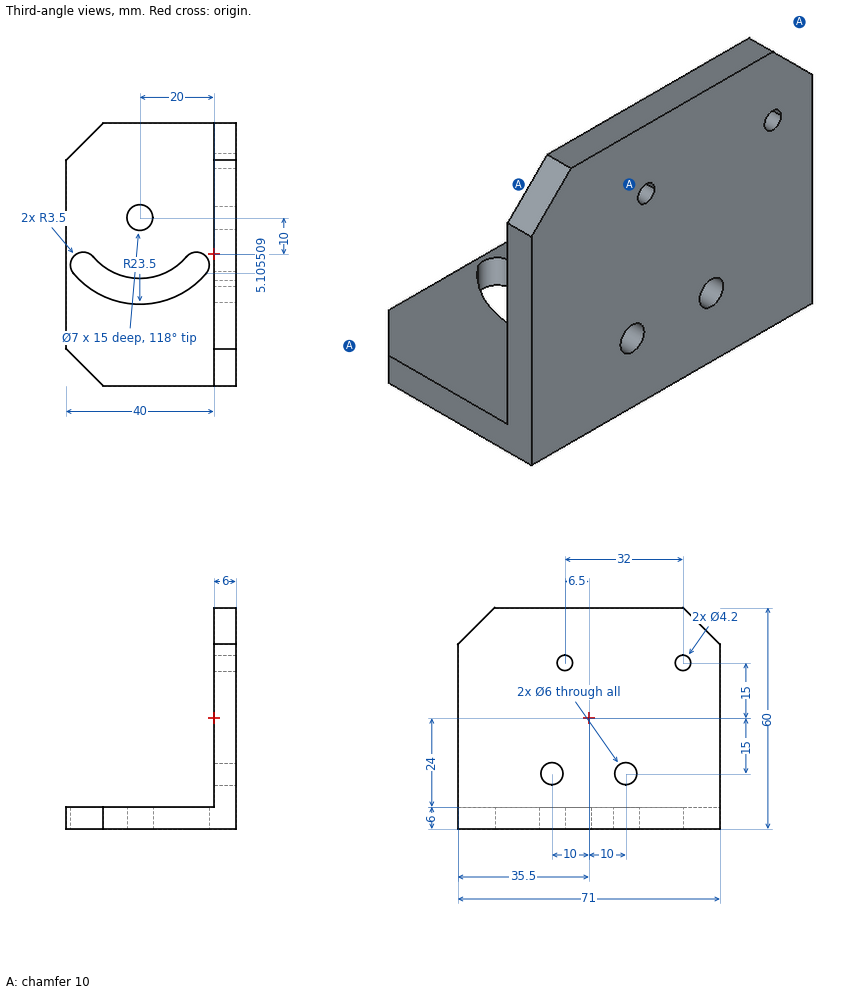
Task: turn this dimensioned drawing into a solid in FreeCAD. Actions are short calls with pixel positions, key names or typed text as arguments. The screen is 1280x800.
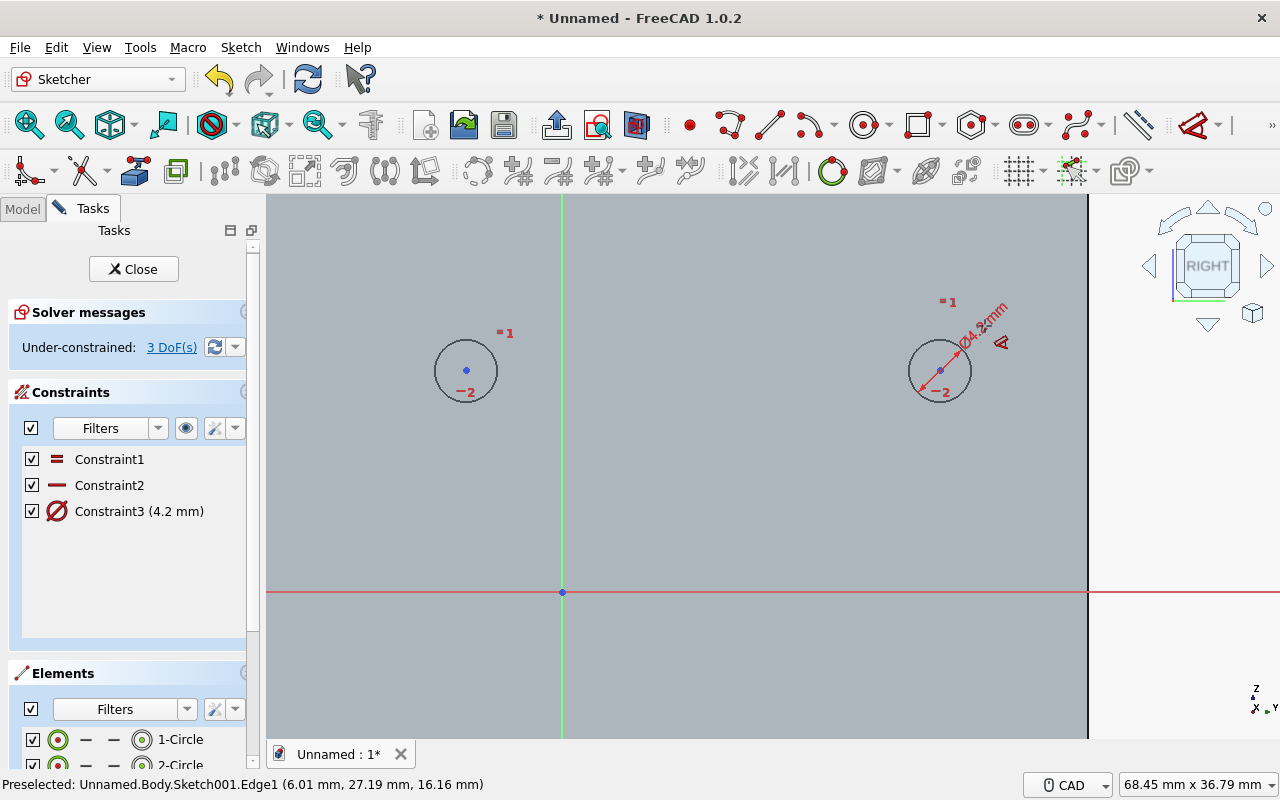
click(940, 371)
click(974, 482)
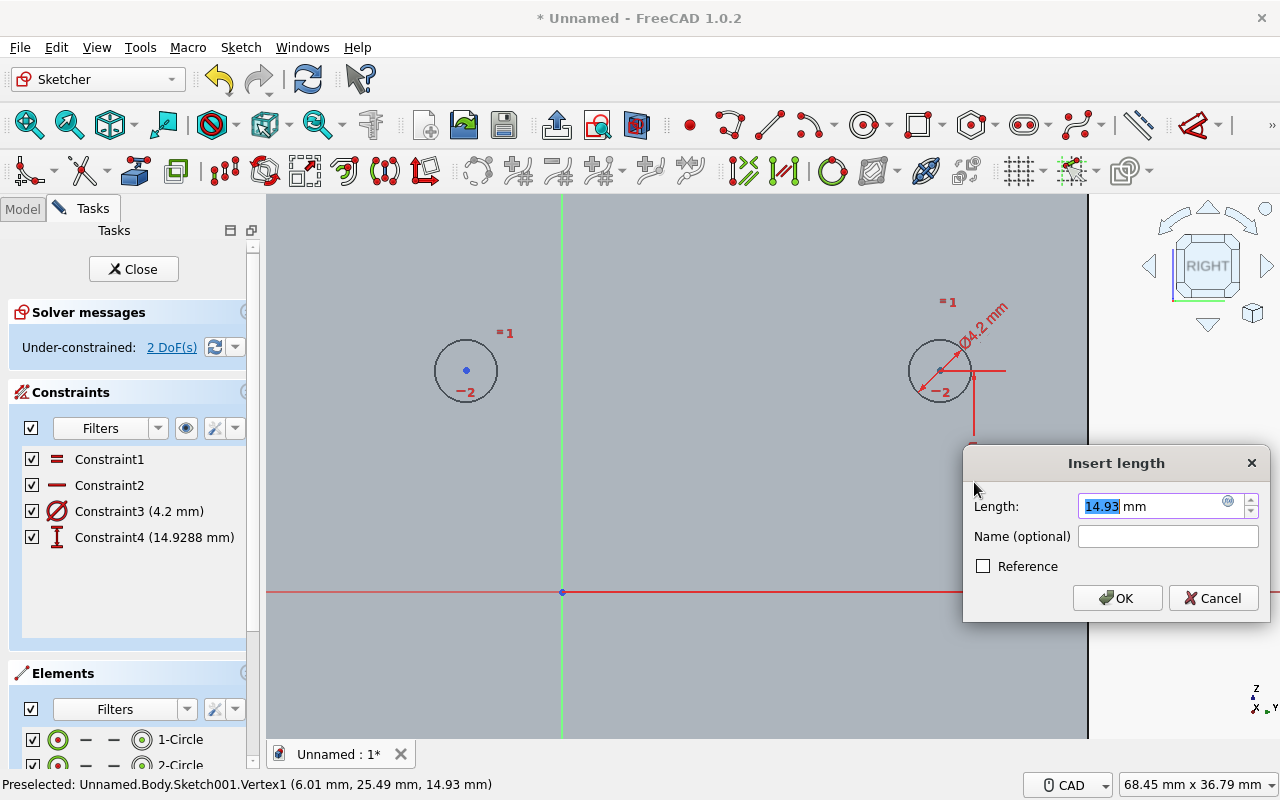
text(15)
key(Return)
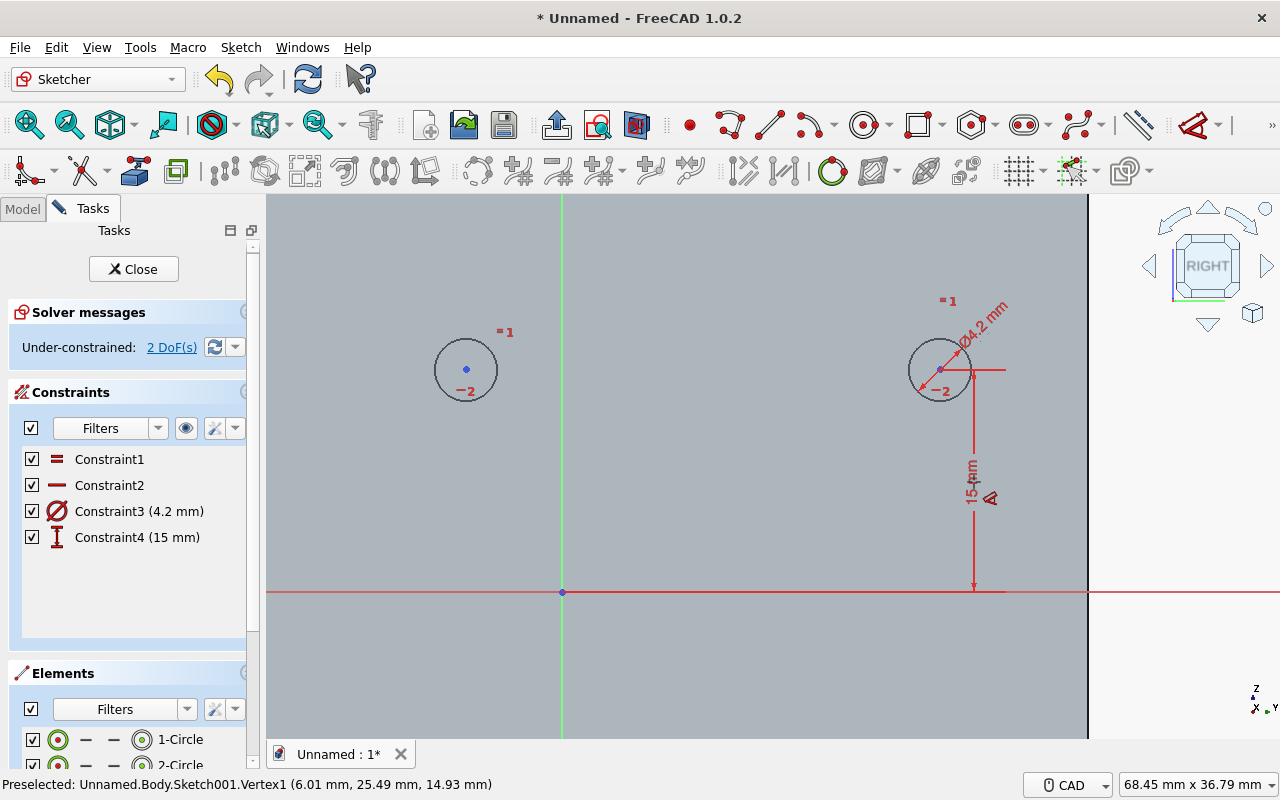
click(466, 370)
click(514, 626)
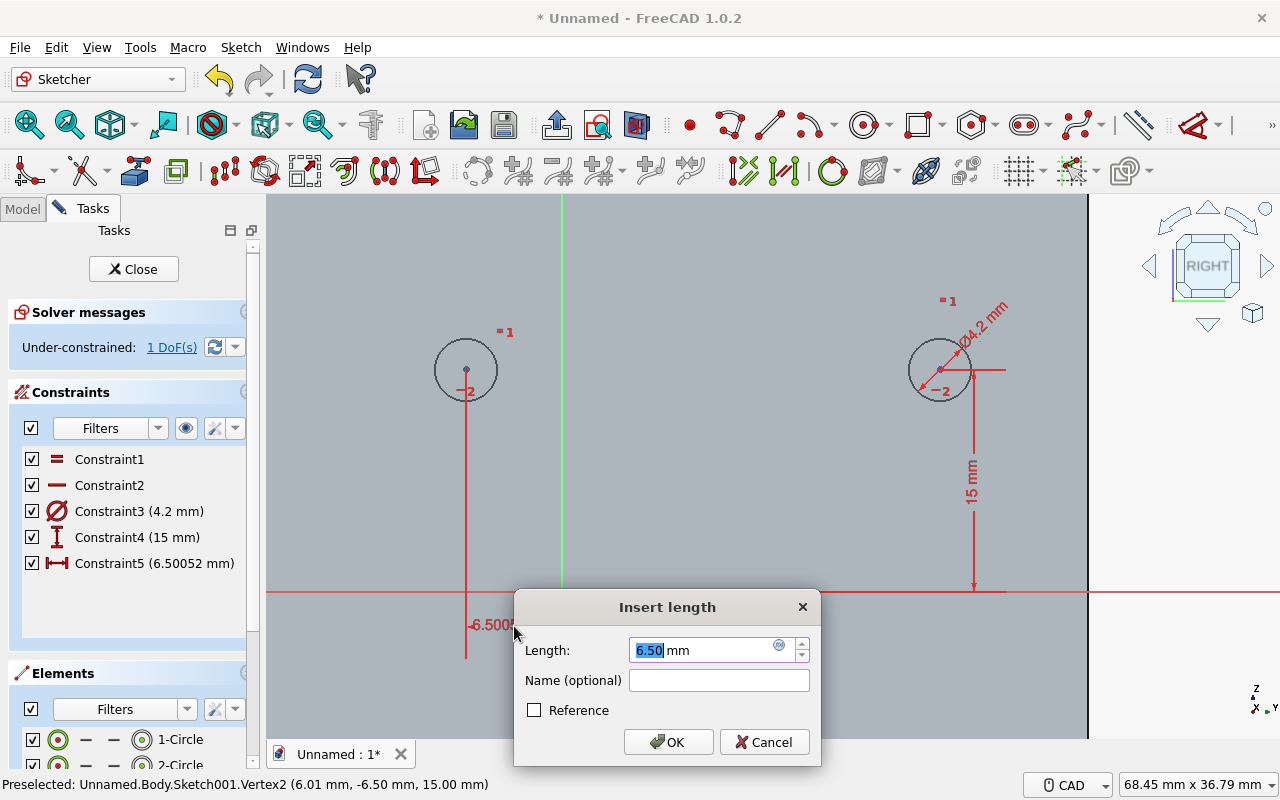
text(6.5)
key(Return)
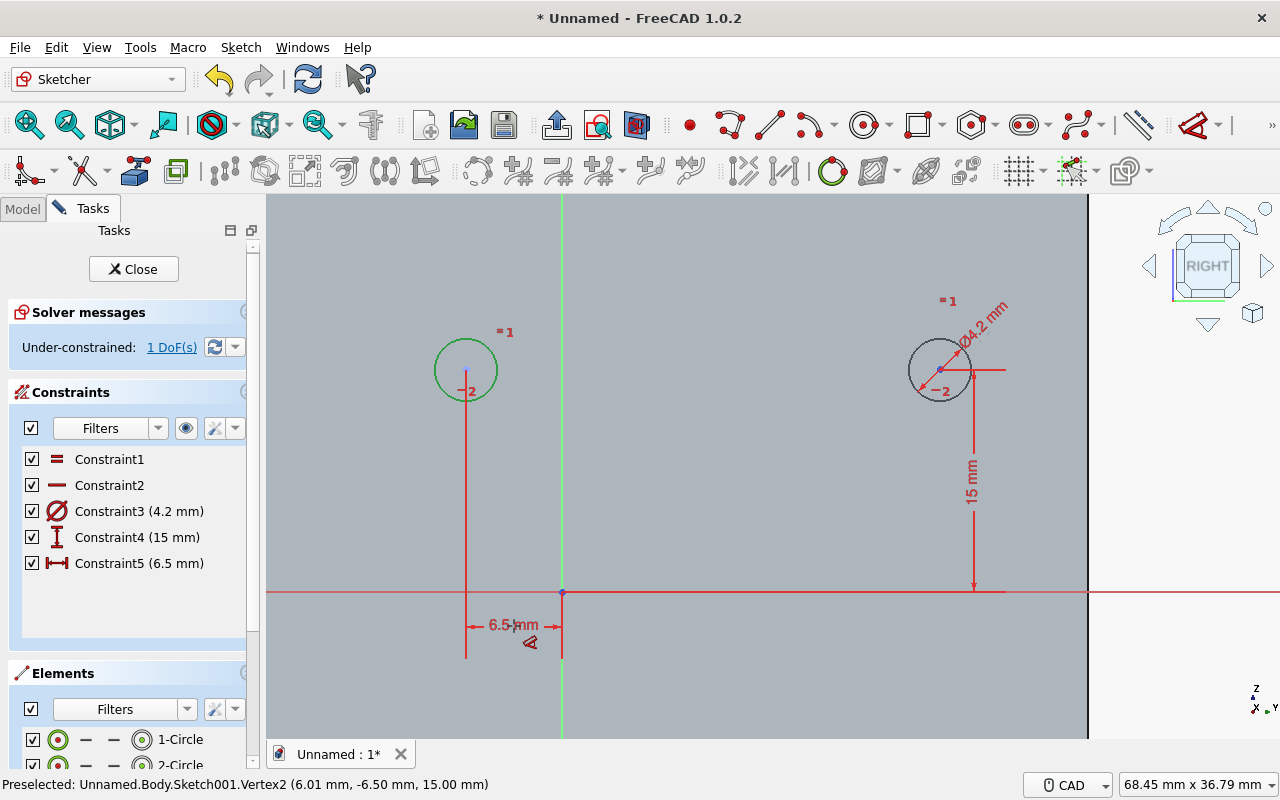
click(940, 370)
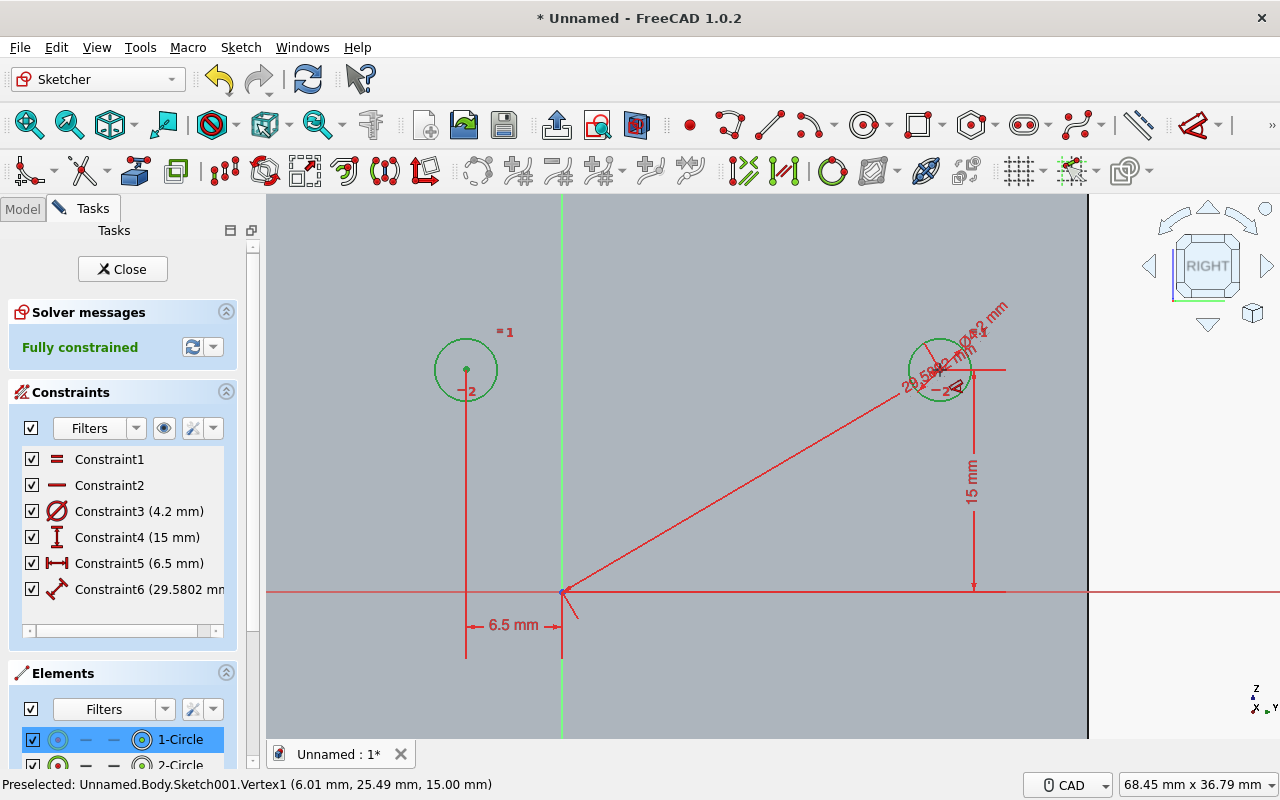
click(466, 370)
click(703, 336)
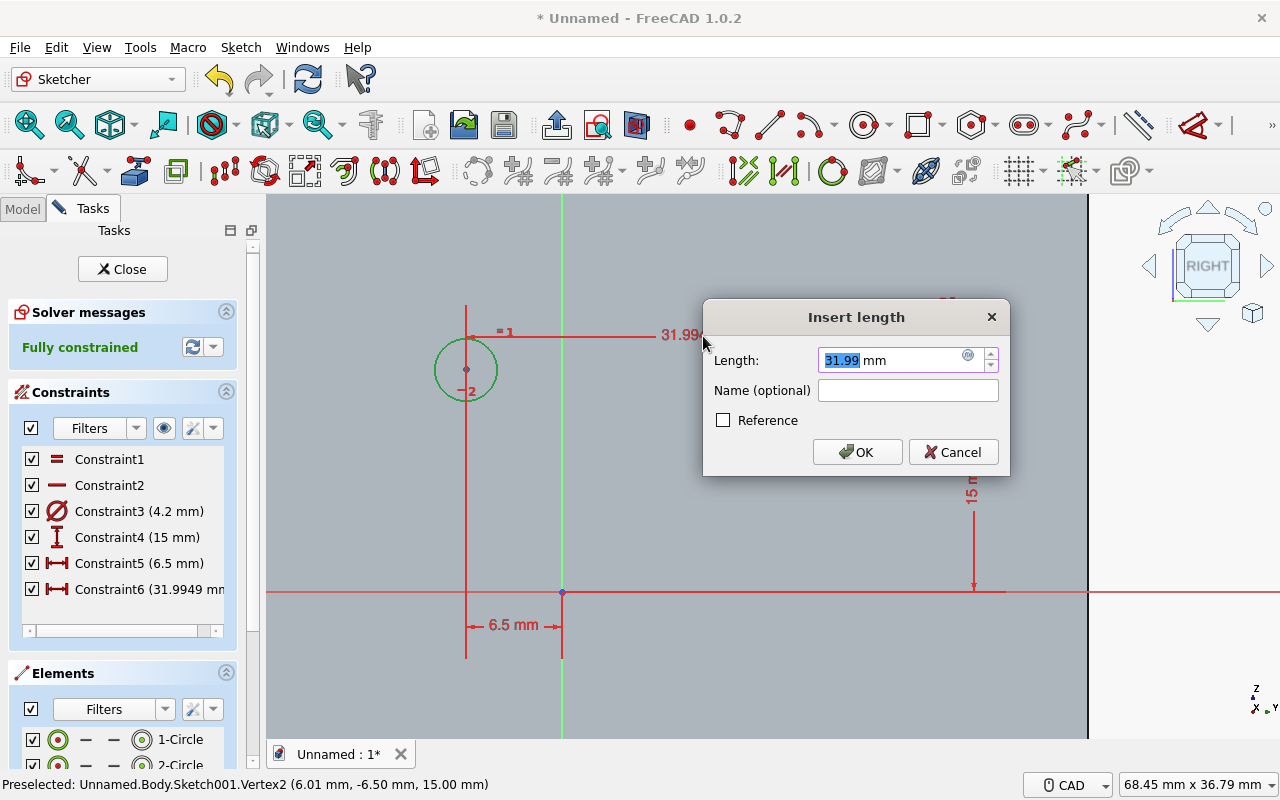
text(32)
key(Return)
key(Escape)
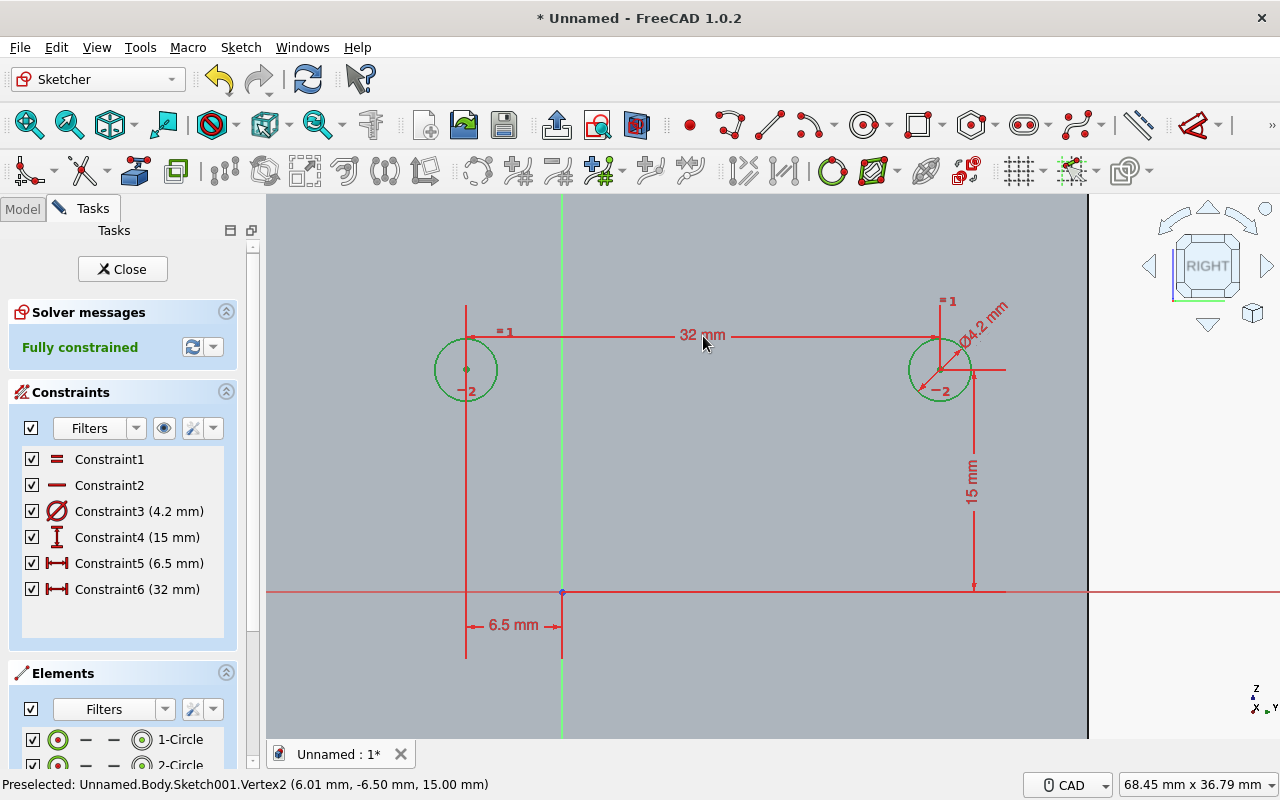
click(123, 269)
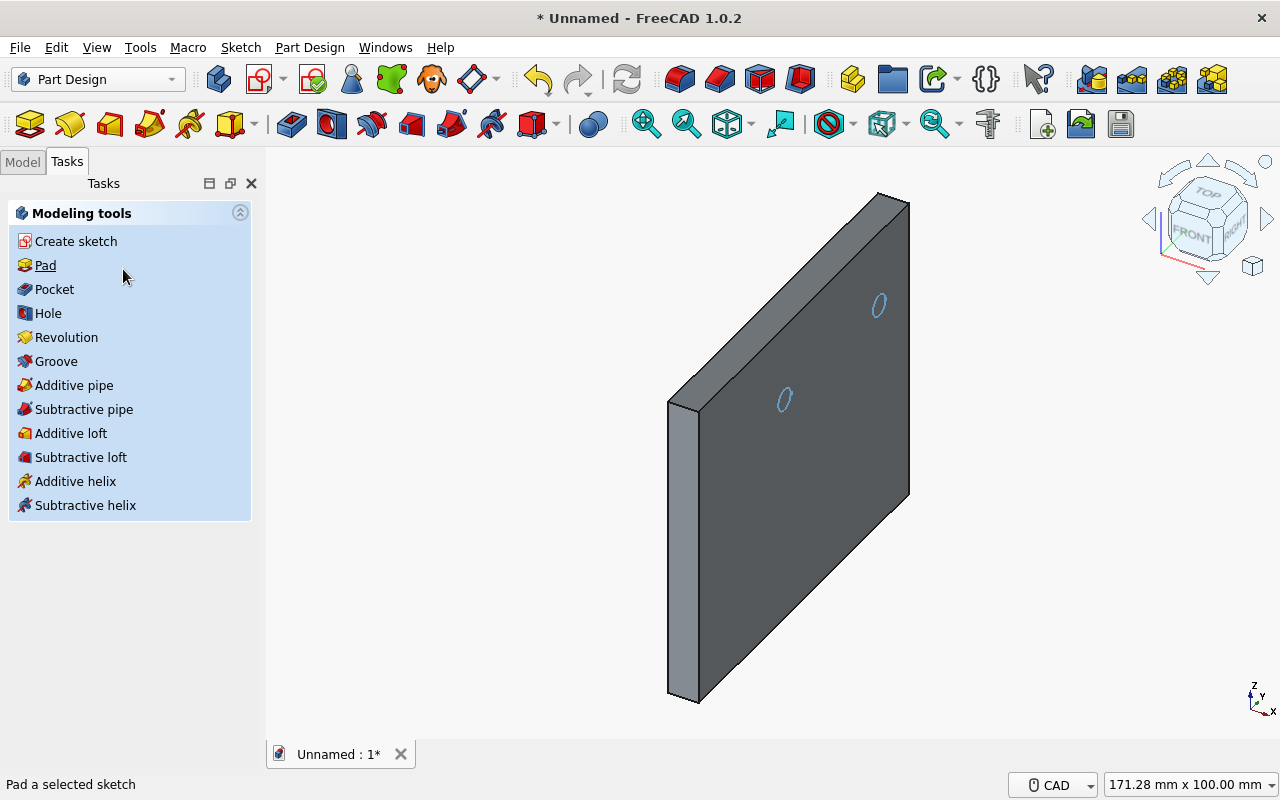
click(292, 124)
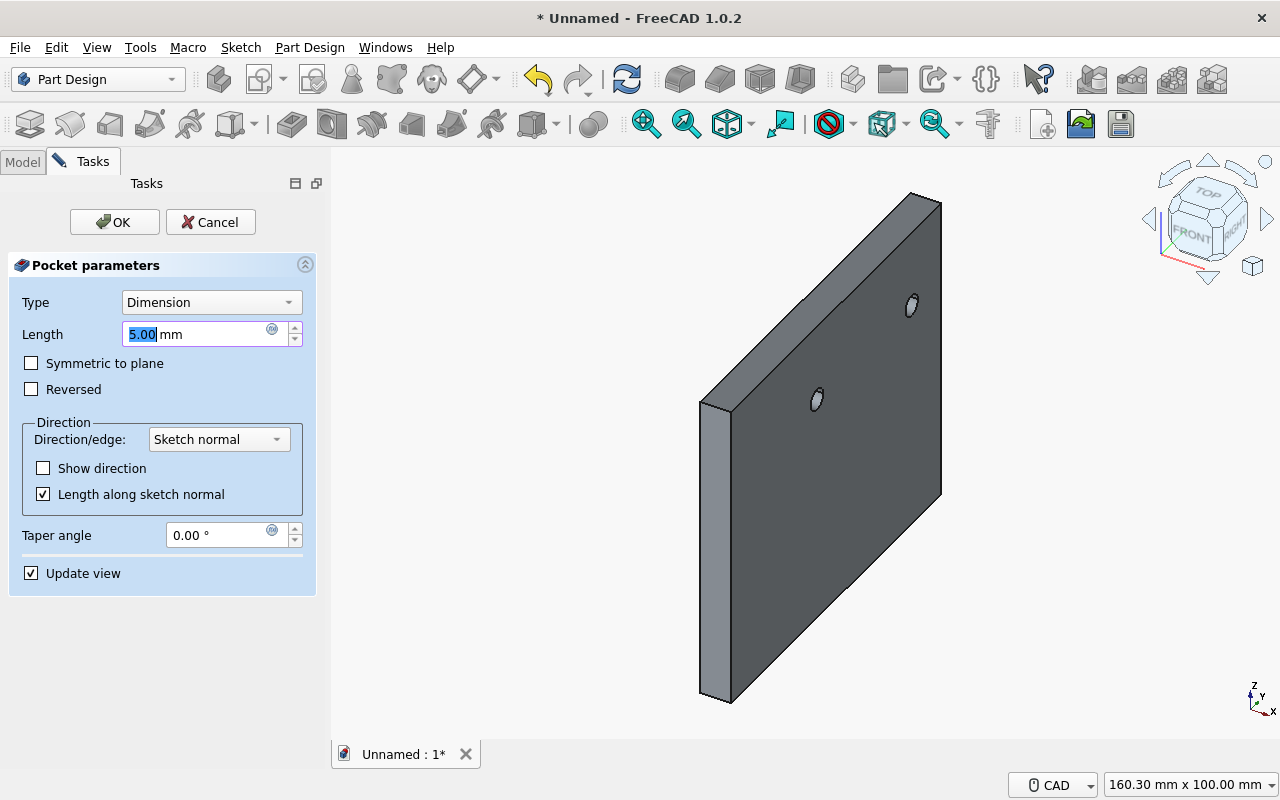
click(212, 302)